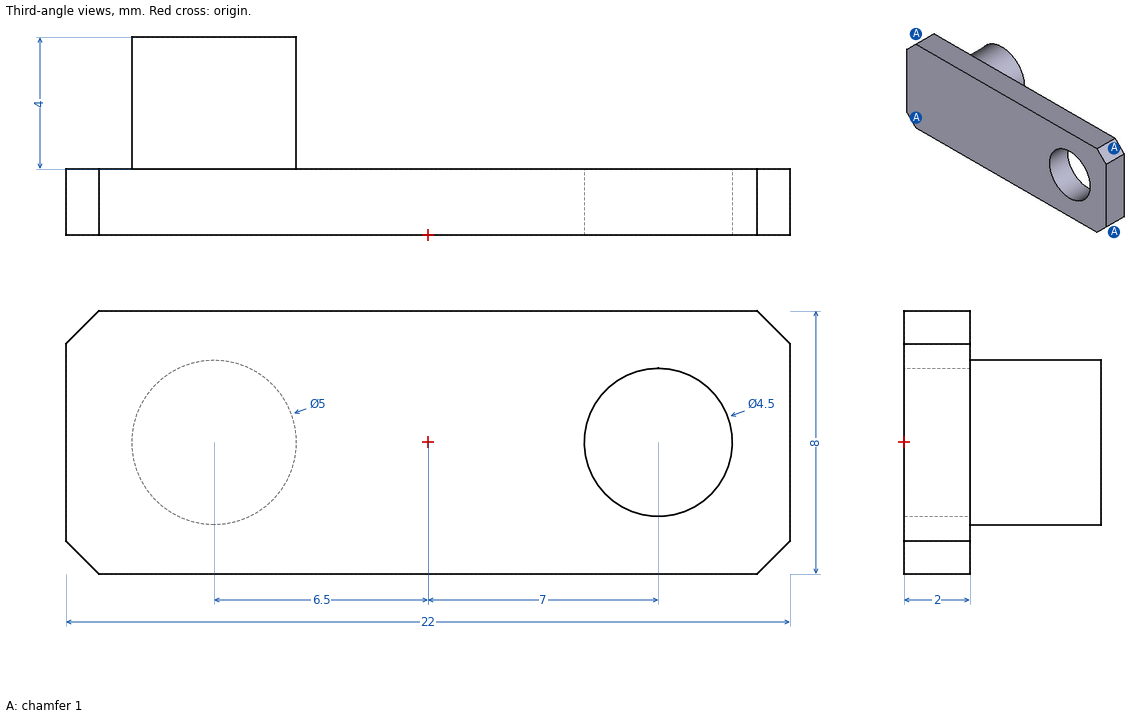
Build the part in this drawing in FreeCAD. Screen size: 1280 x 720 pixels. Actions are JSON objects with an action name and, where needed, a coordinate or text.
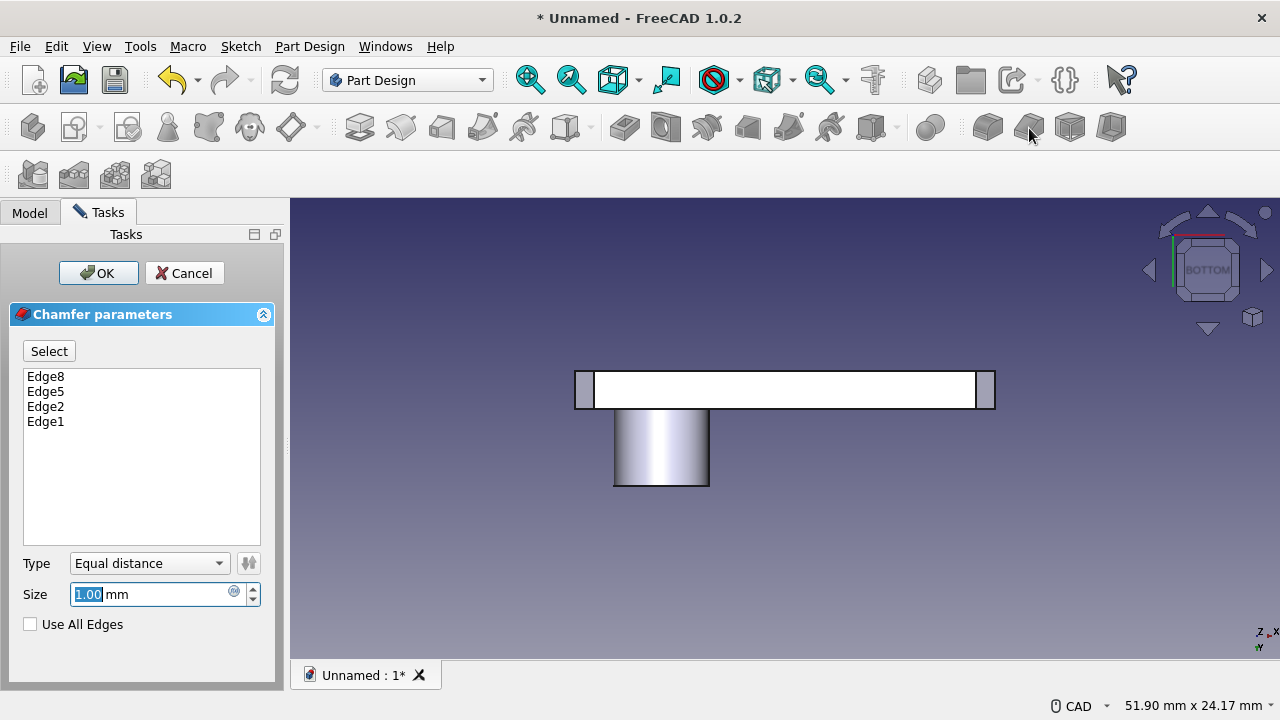
{"action": "type", "text": "1"}
{"action": "key", "text": "Tab"}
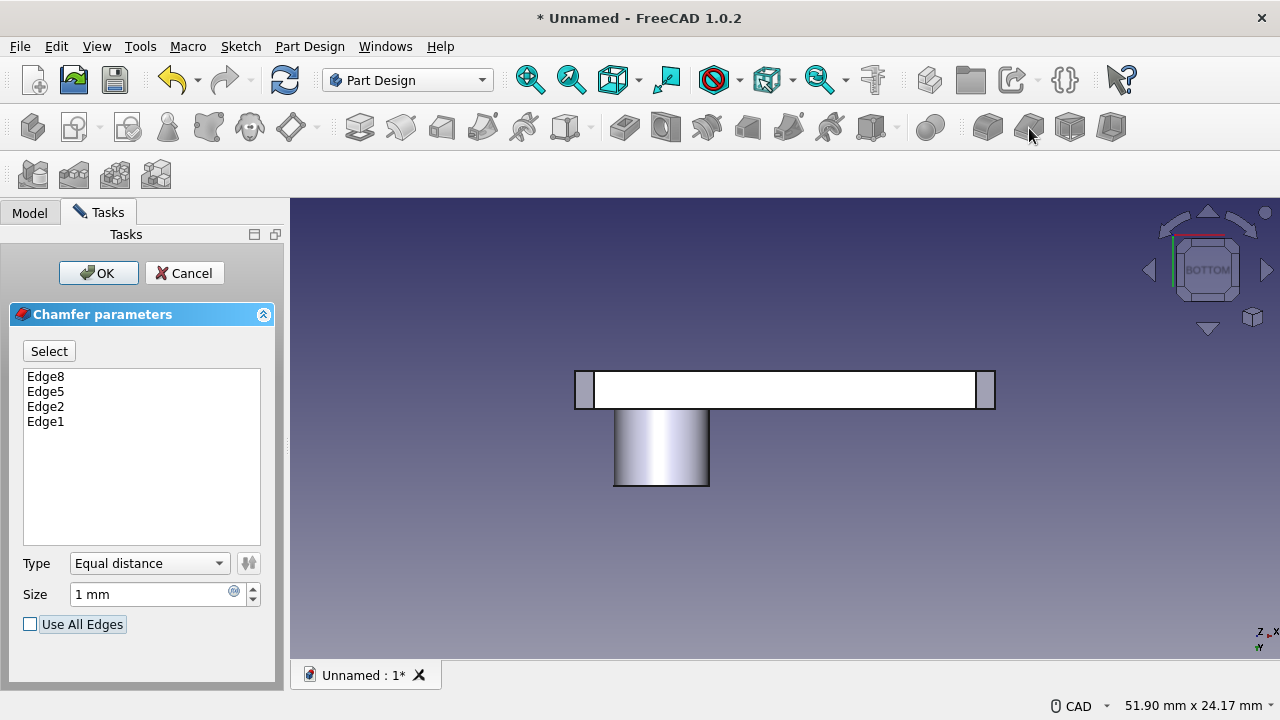
{"action": "left_click", "coordinate": [99, 273]}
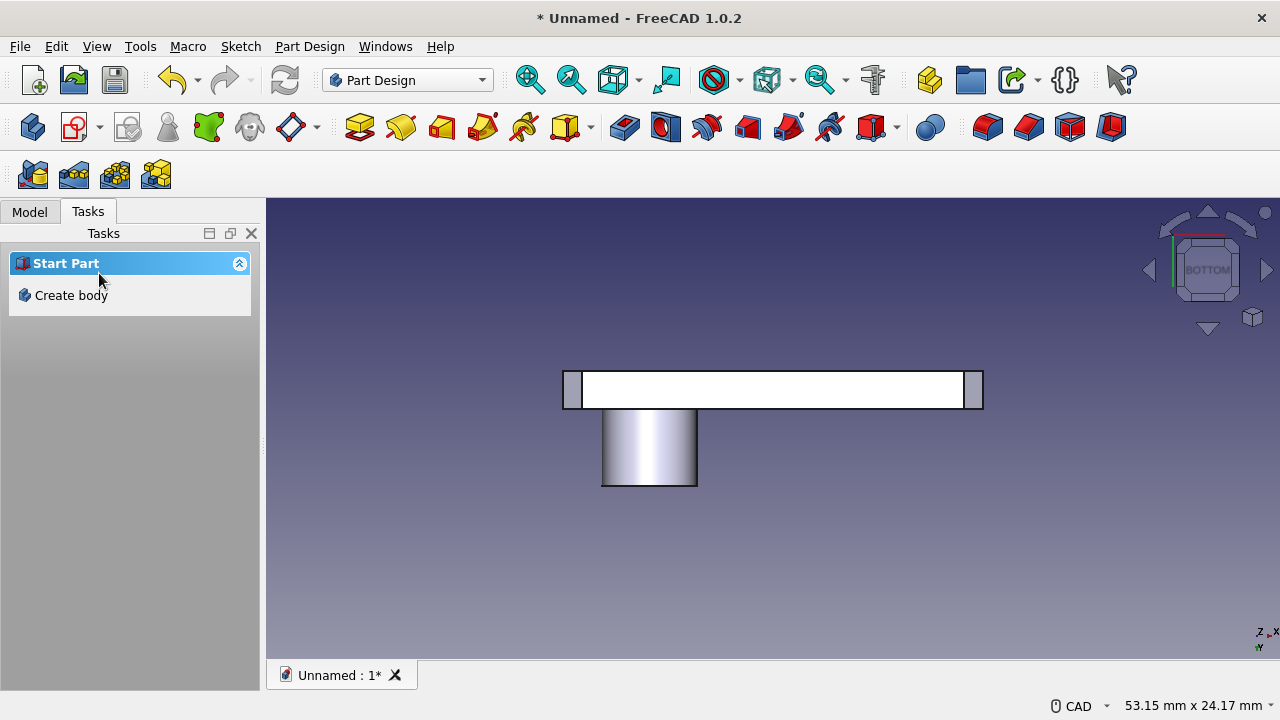
{"action": "key", "text": "0"}